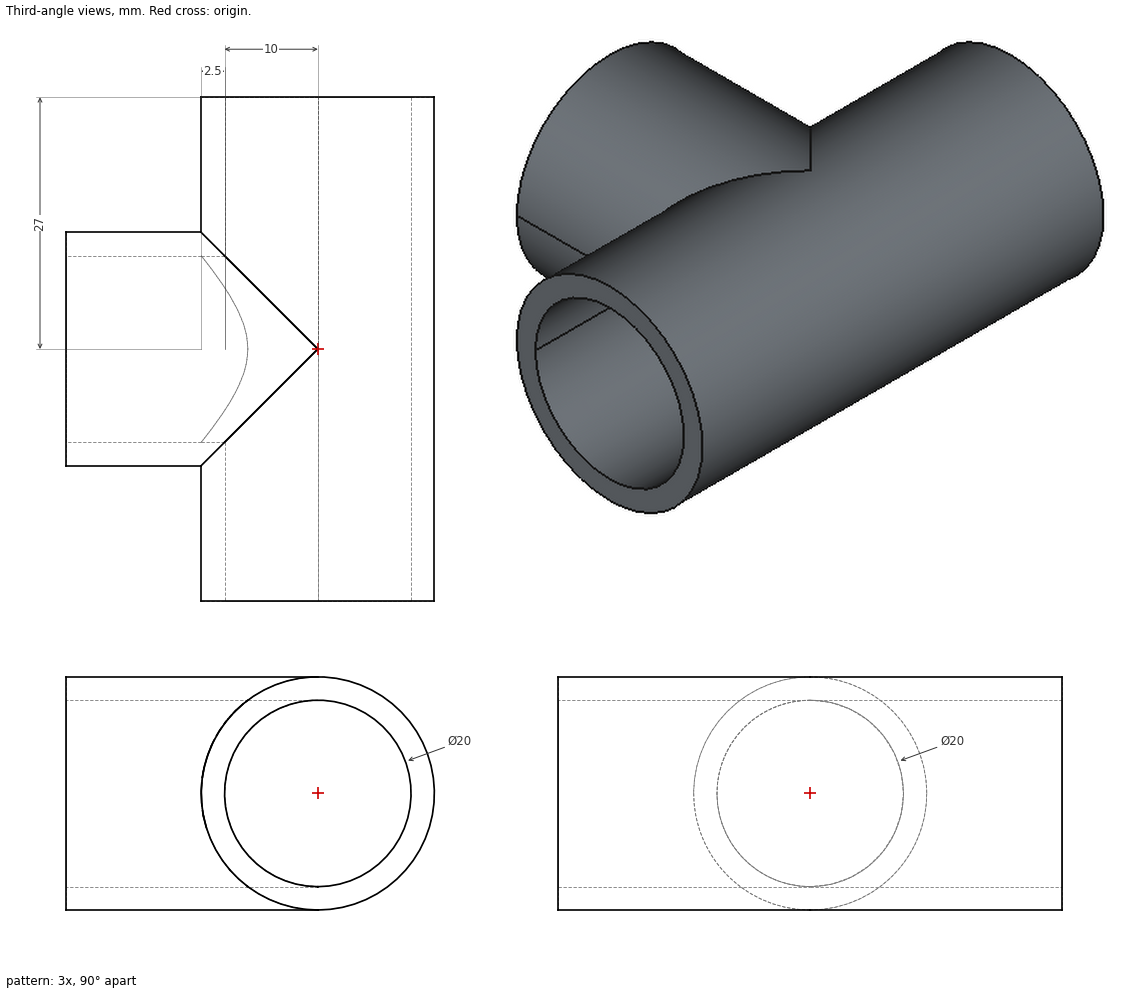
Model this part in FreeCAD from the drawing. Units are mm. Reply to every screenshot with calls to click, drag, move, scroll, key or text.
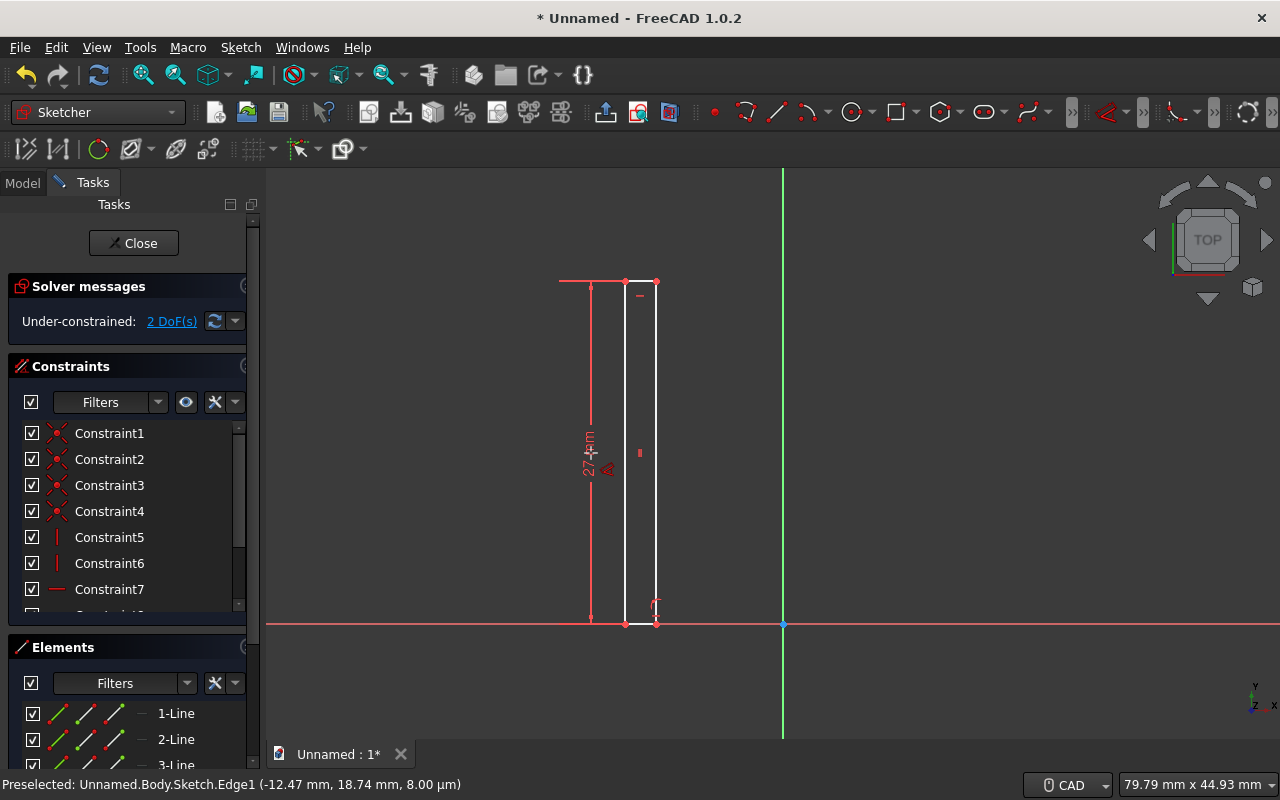
scroll(634, 624, up, 2)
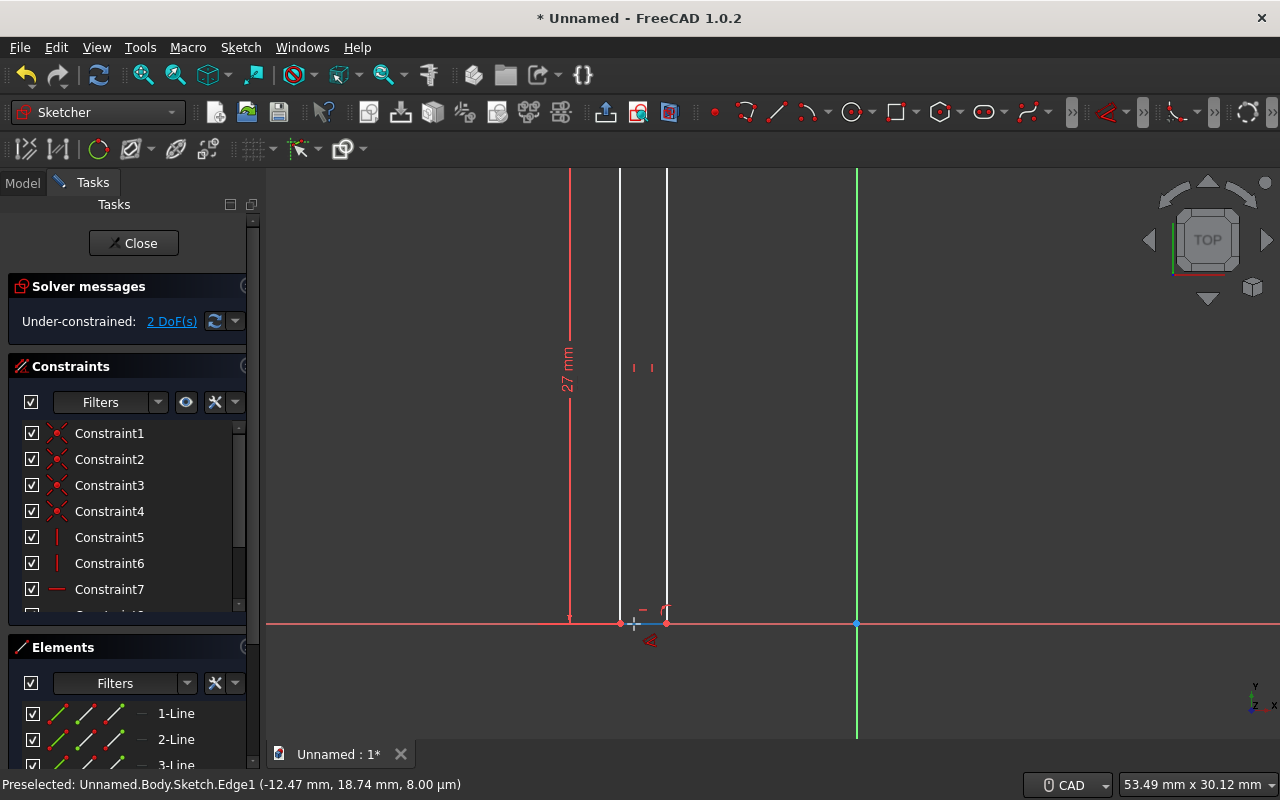
click(634, 624)
click(644, 658)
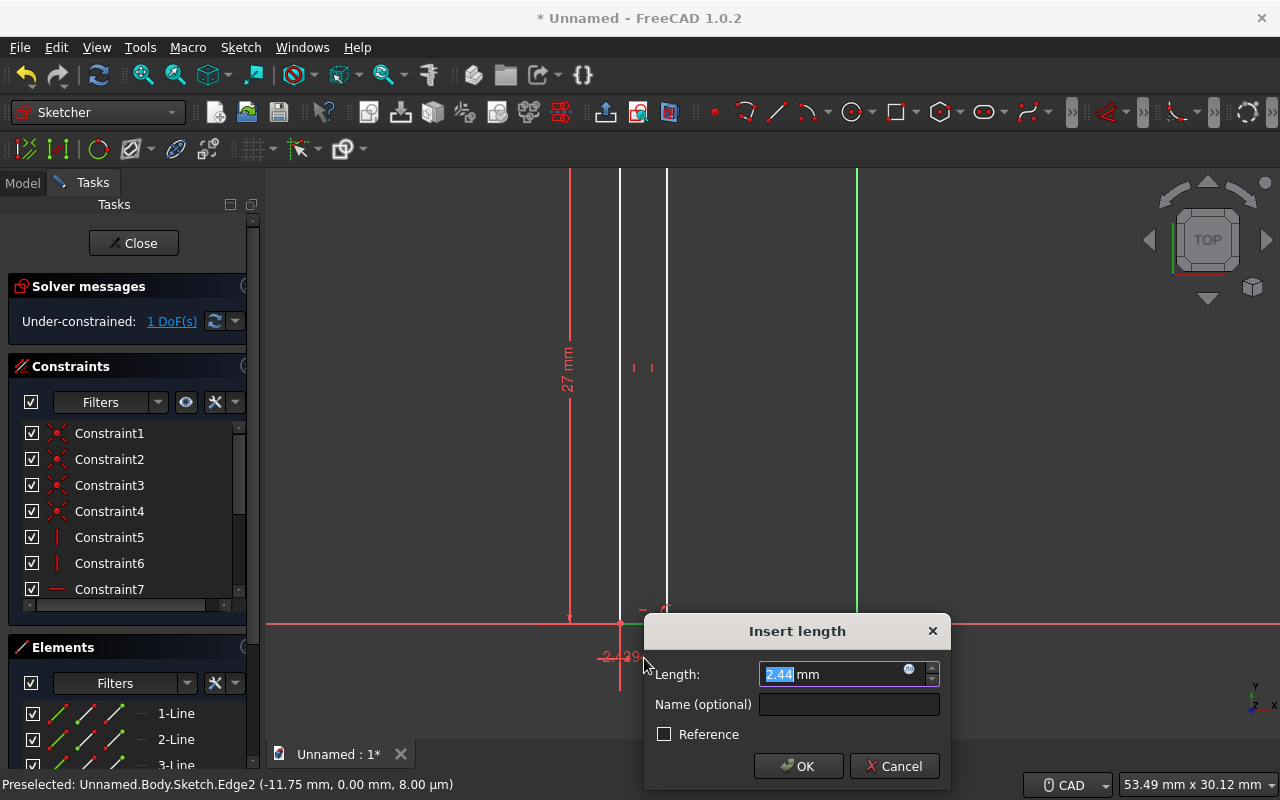
text(2.5)
key(Return)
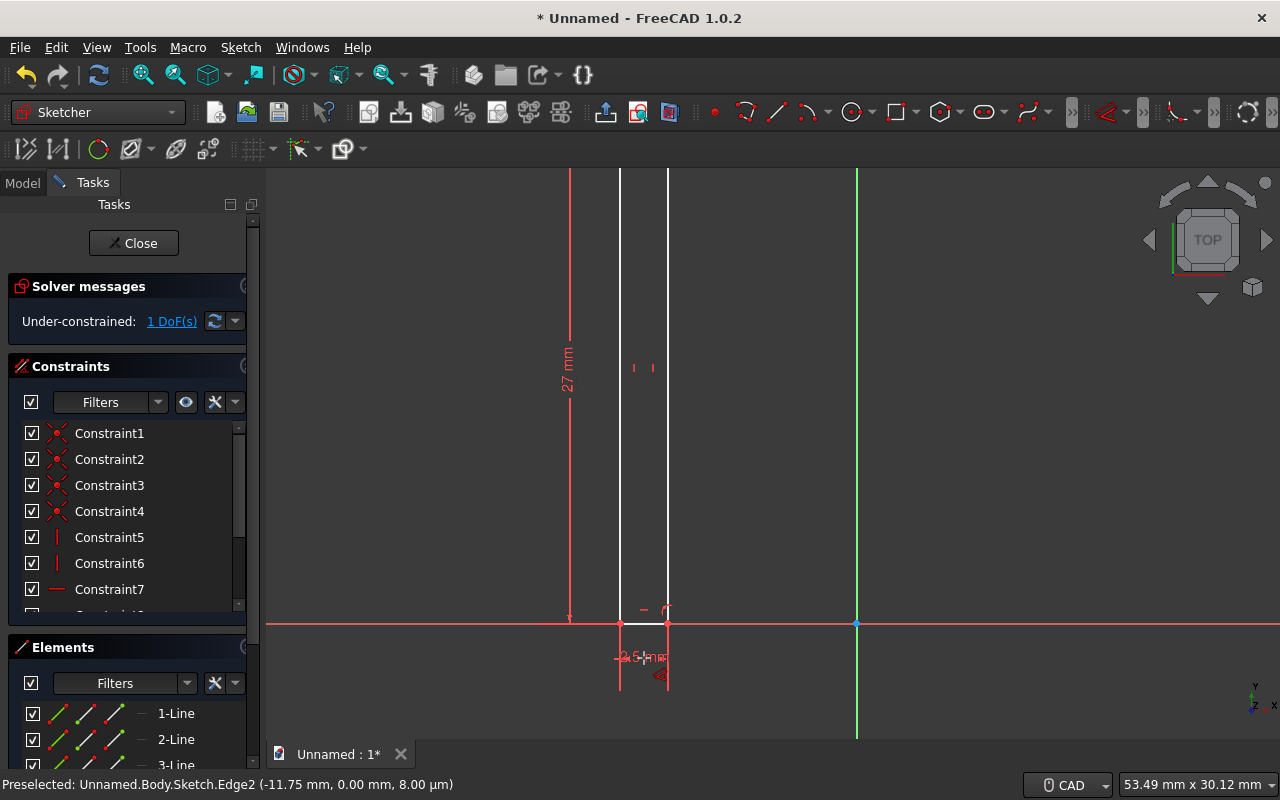
click(668, 624)
click(762, 658)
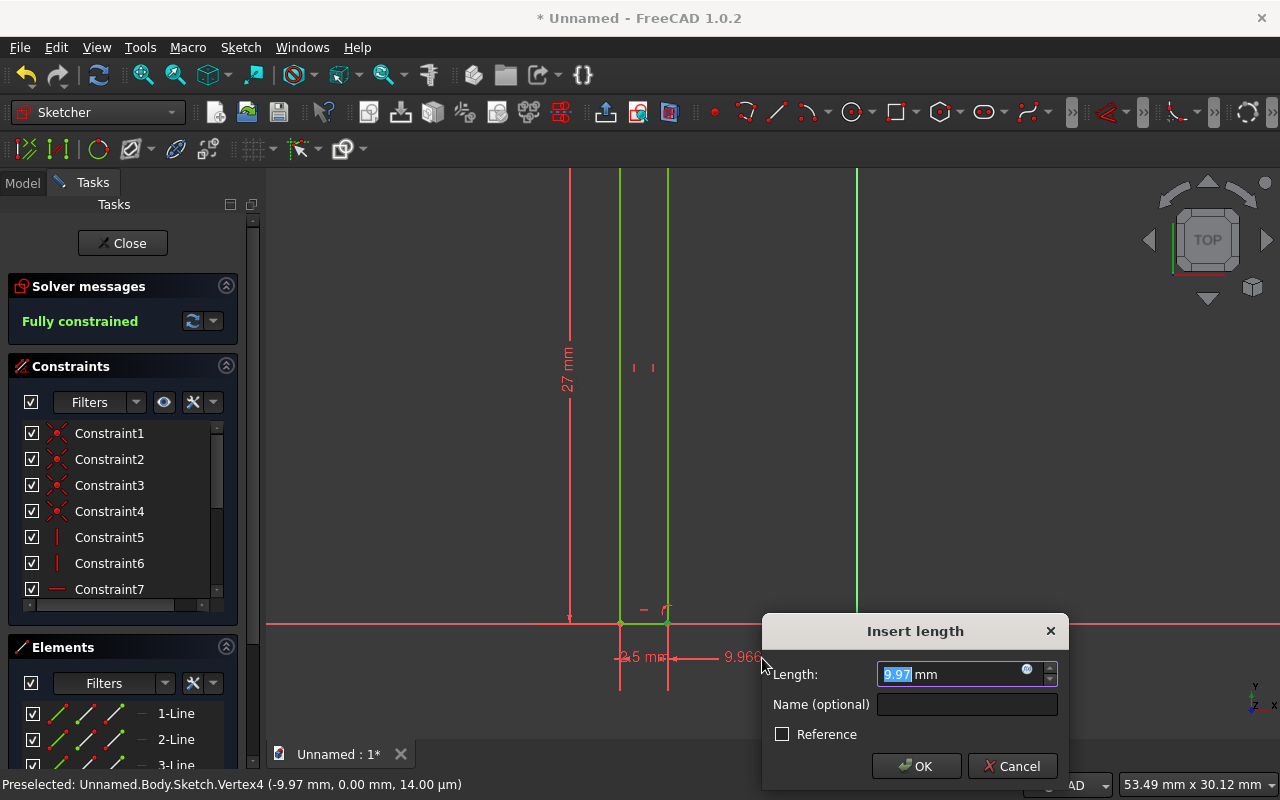
text(10)
key(Return)
key(Escape)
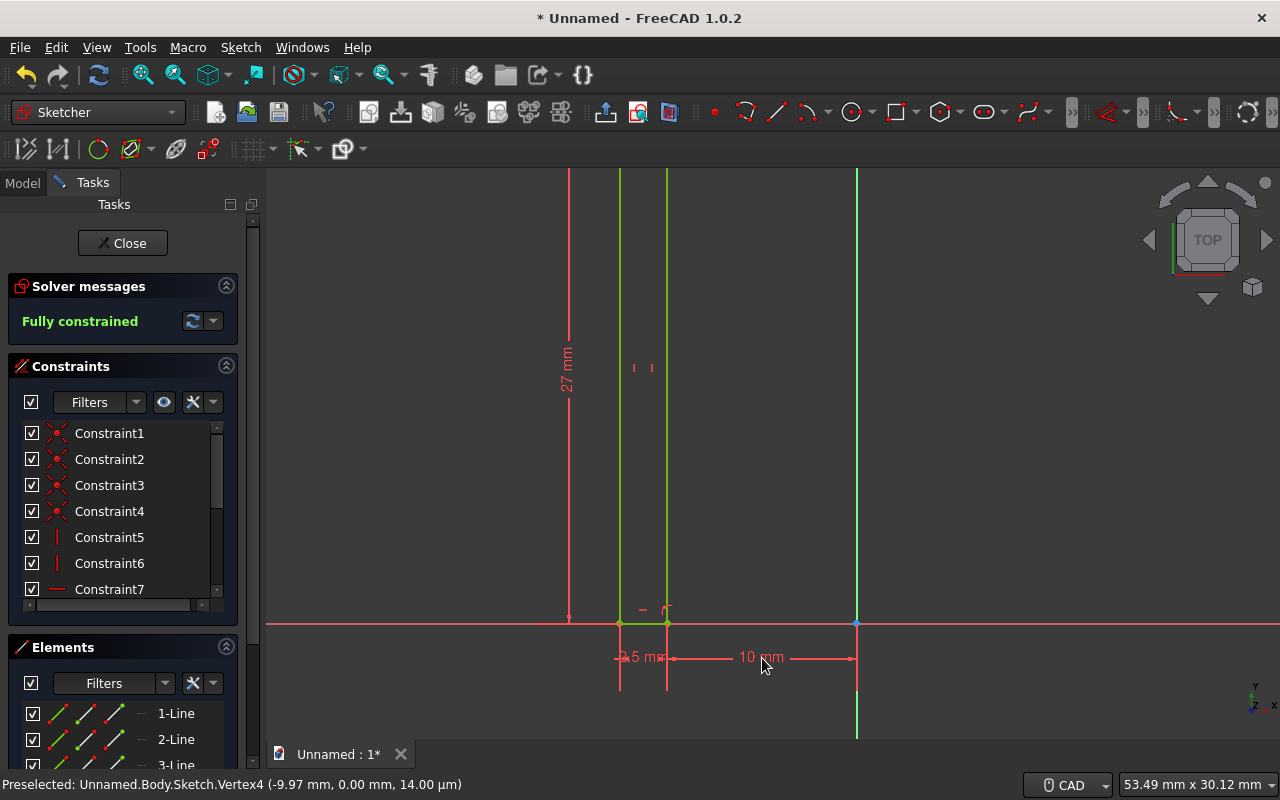
click(123, 243)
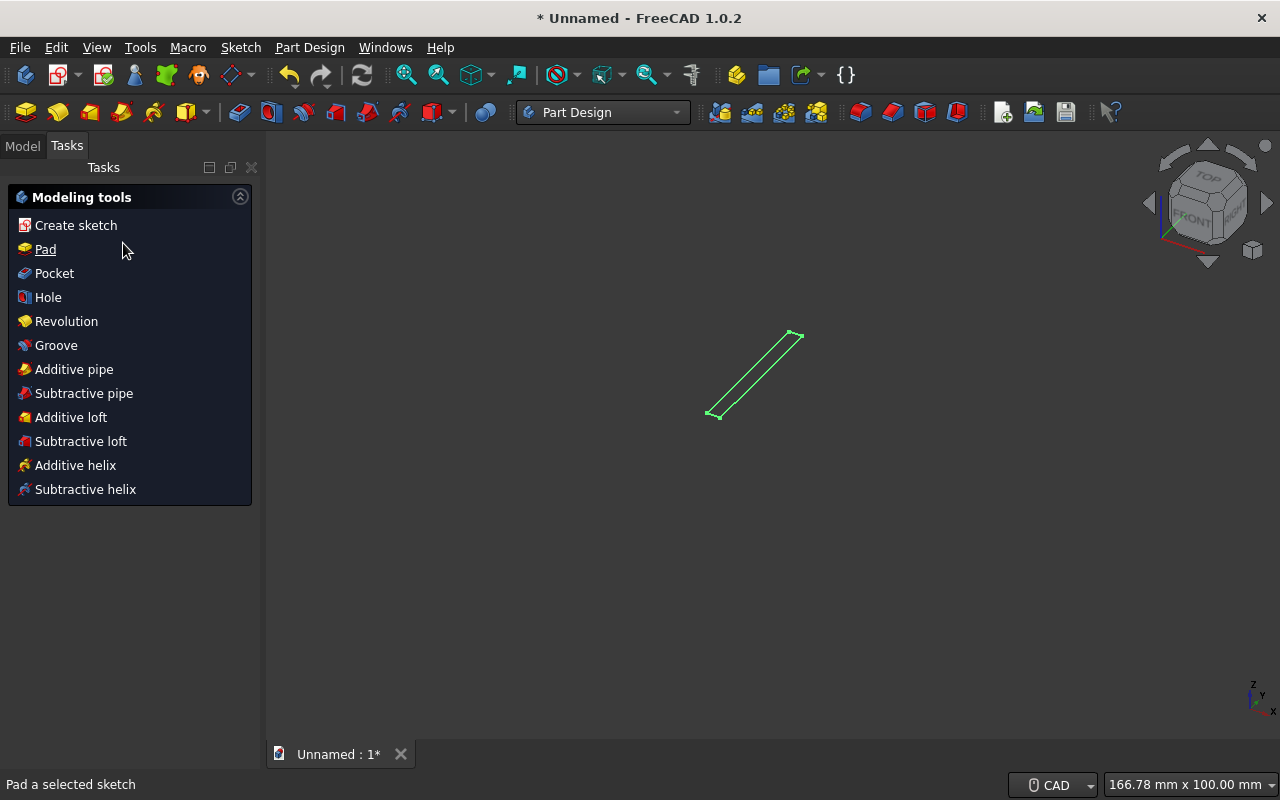
click(58, 112)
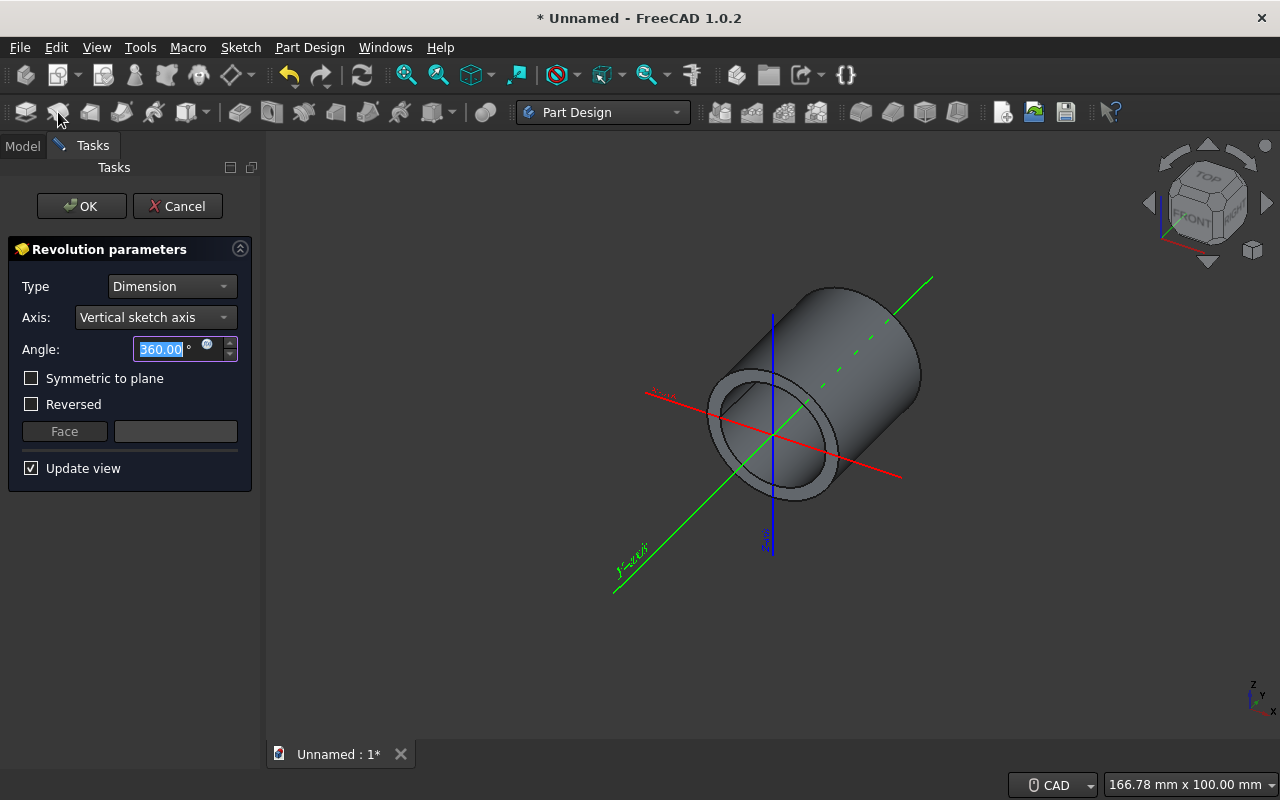
click(82, 206)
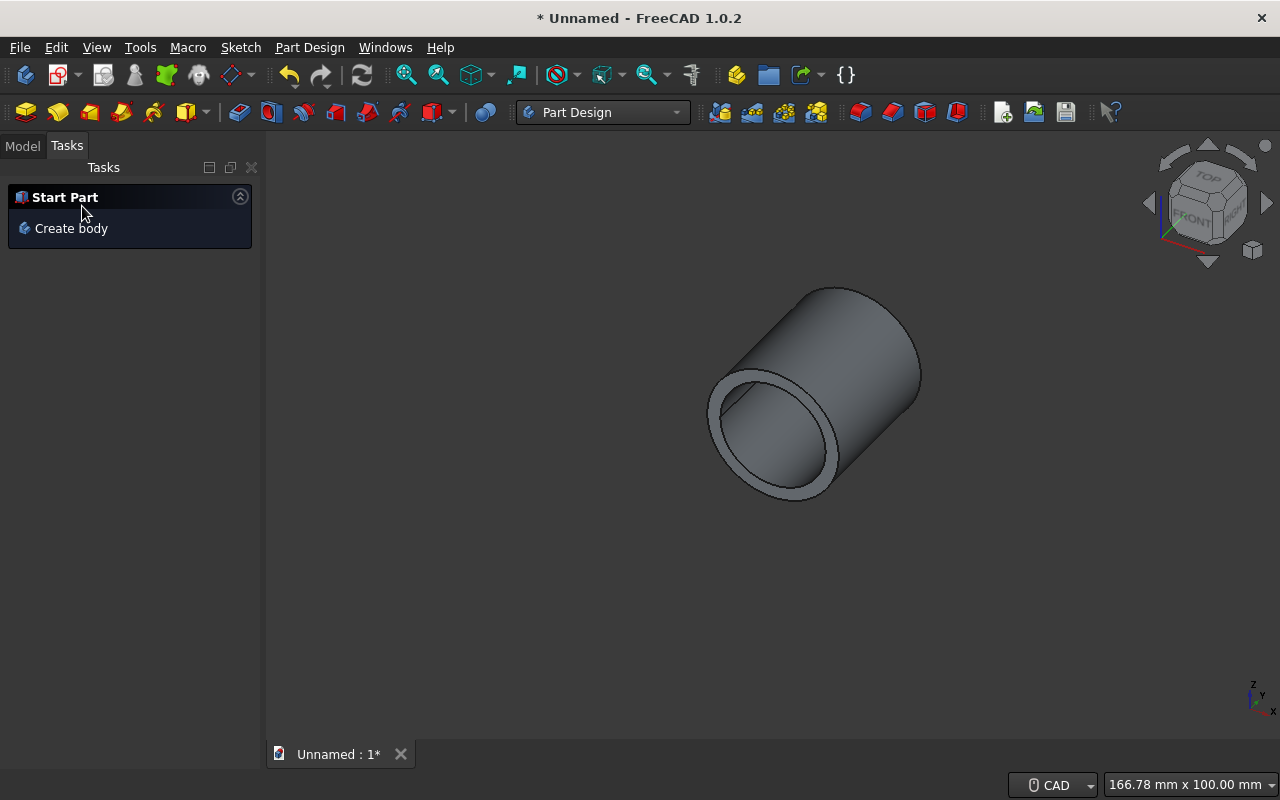
key(v)
key(f)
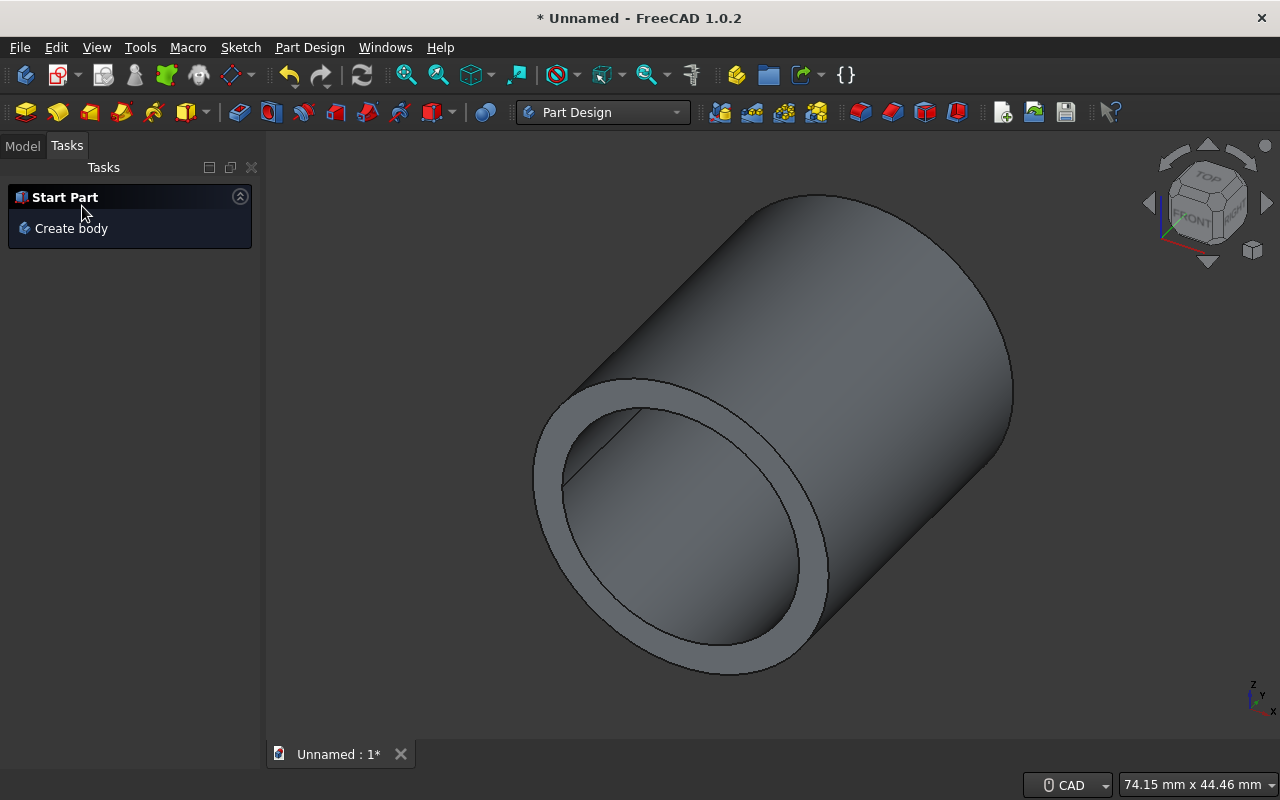
click(23, 145)